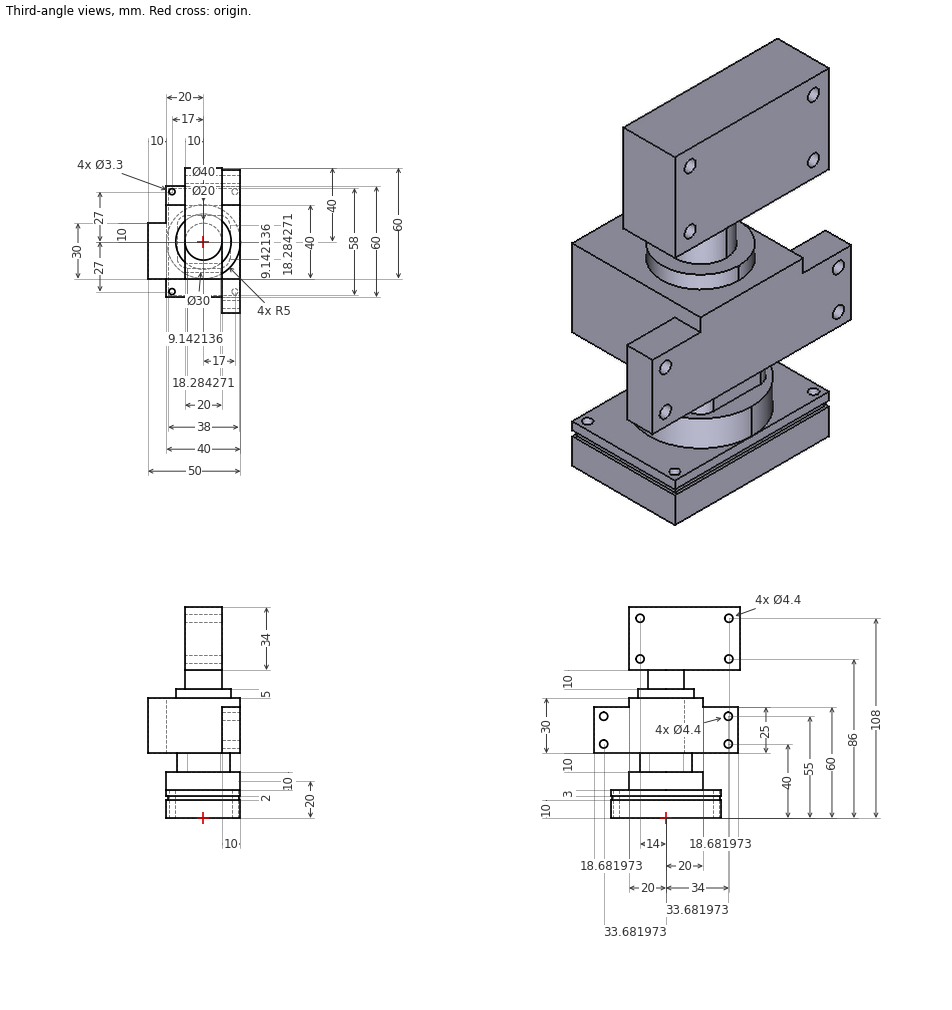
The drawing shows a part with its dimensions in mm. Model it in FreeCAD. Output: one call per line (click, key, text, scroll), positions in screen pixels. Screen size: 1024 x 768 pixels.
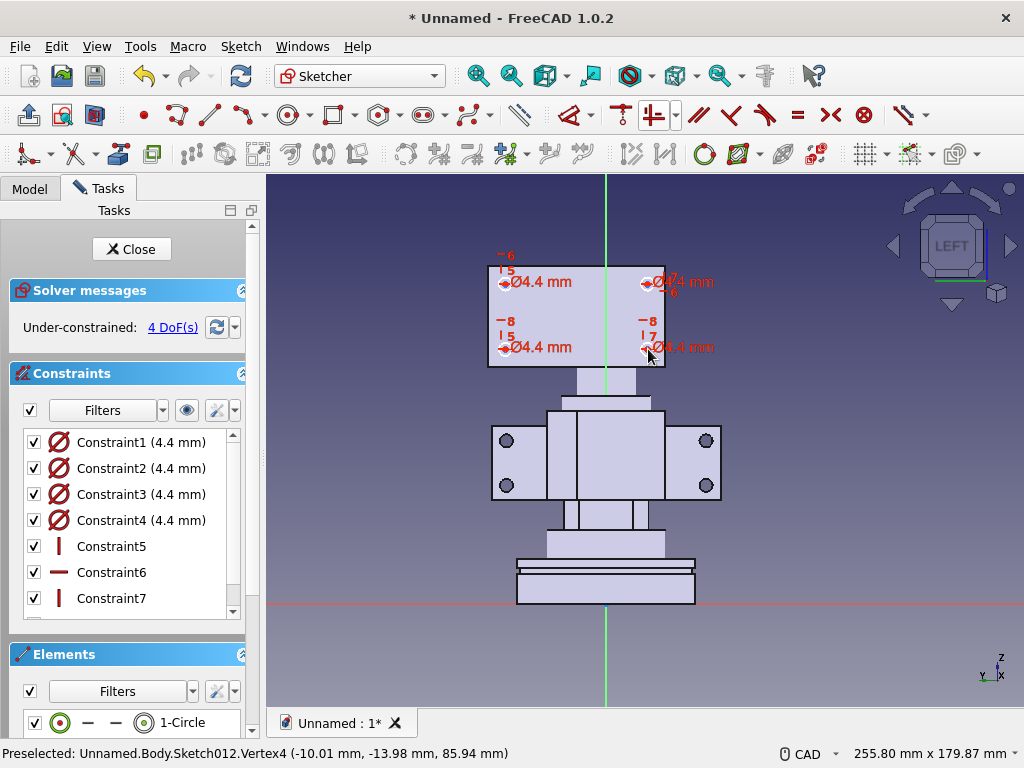
click(568, 116)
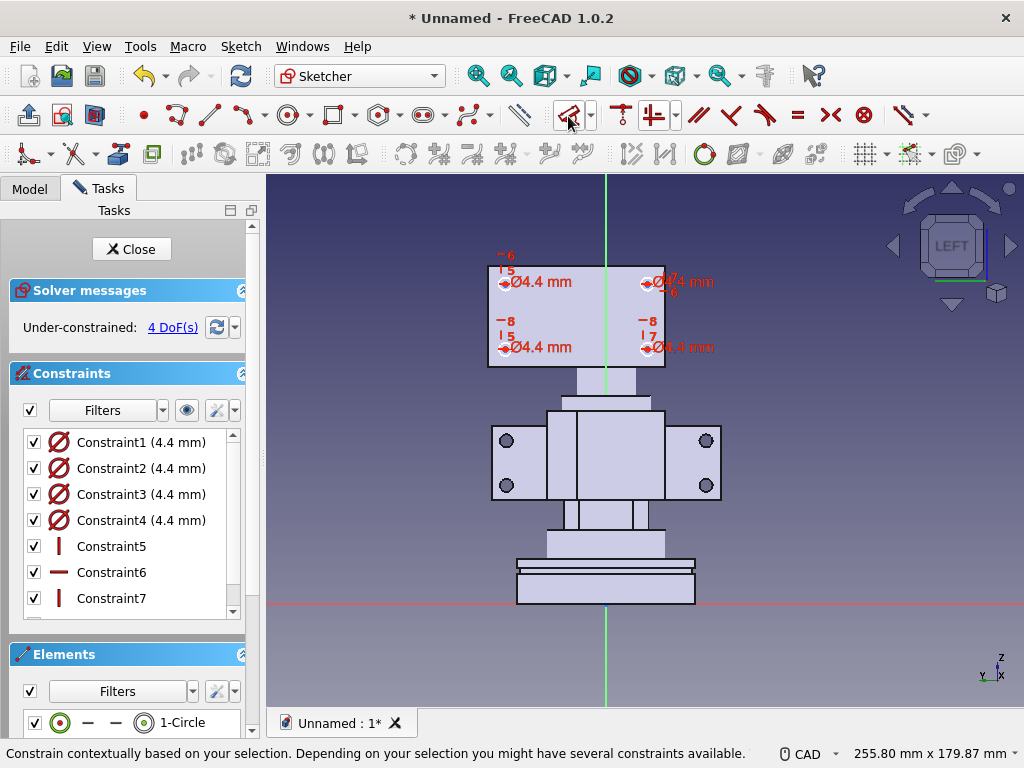
click(505, 284)
click(556, 638)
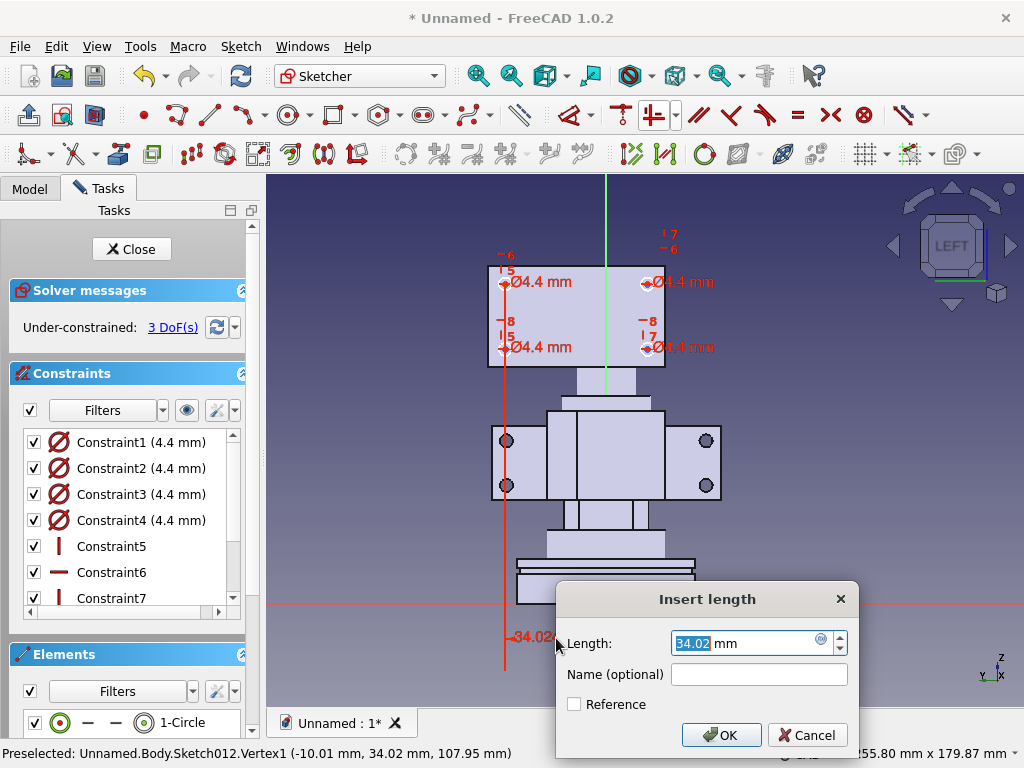
text(34)
key(Return)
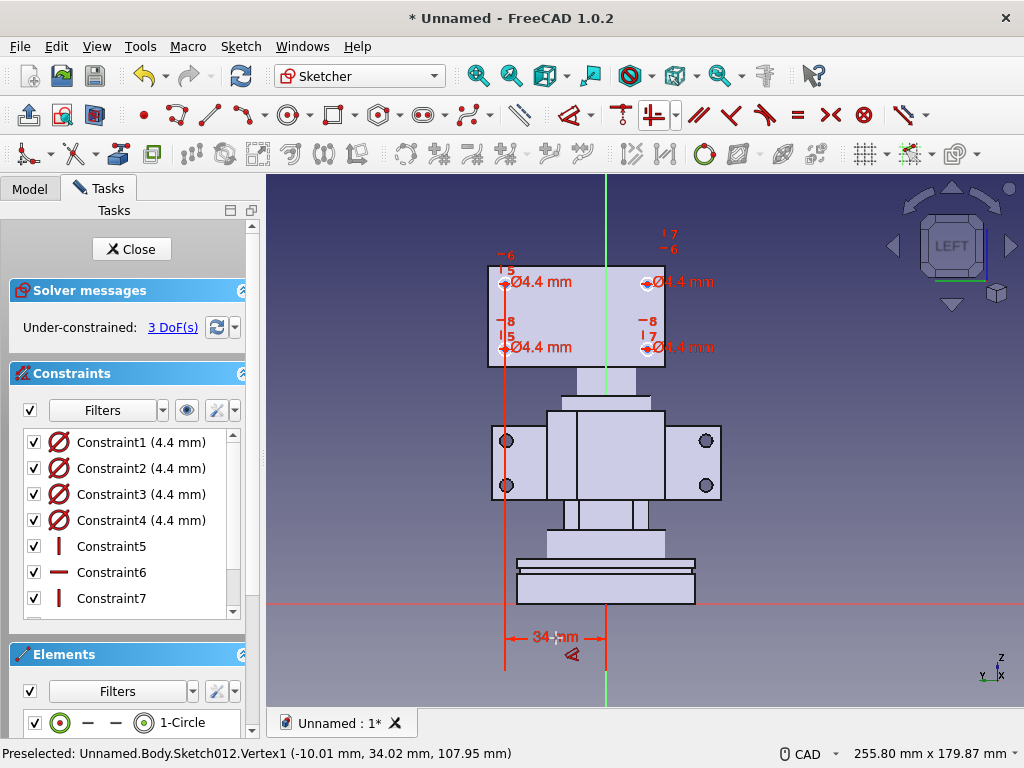
click(505, 349)
click(471, 477)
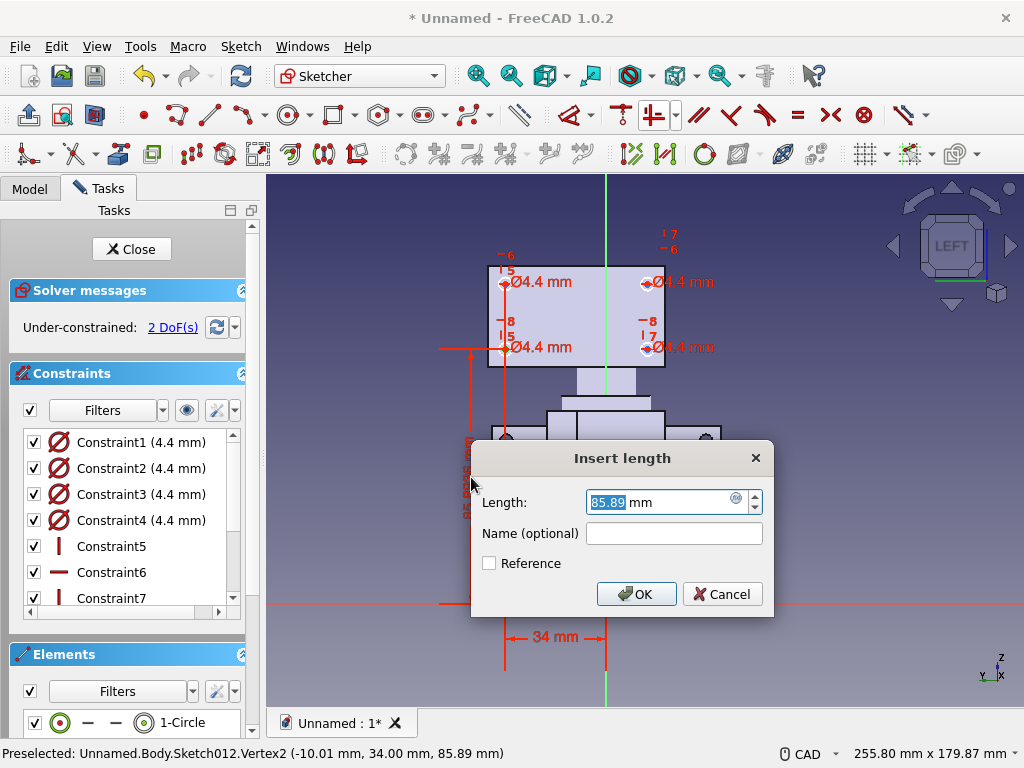
text(86)
key(Return)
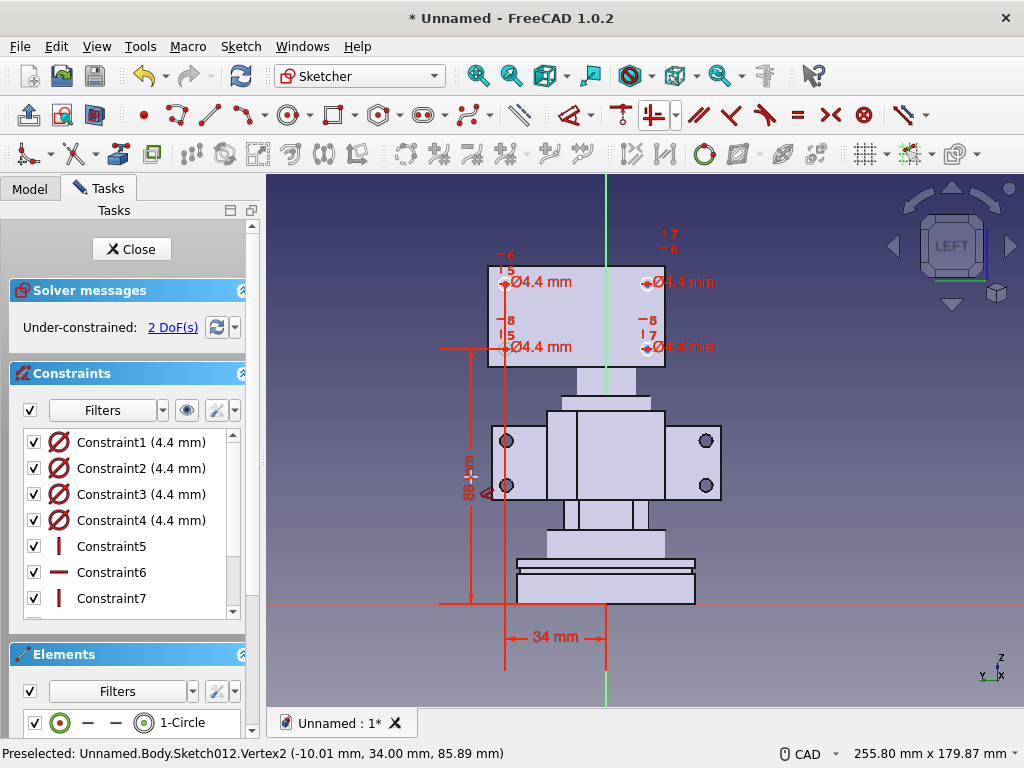
click(648, 284)
click(627, 638)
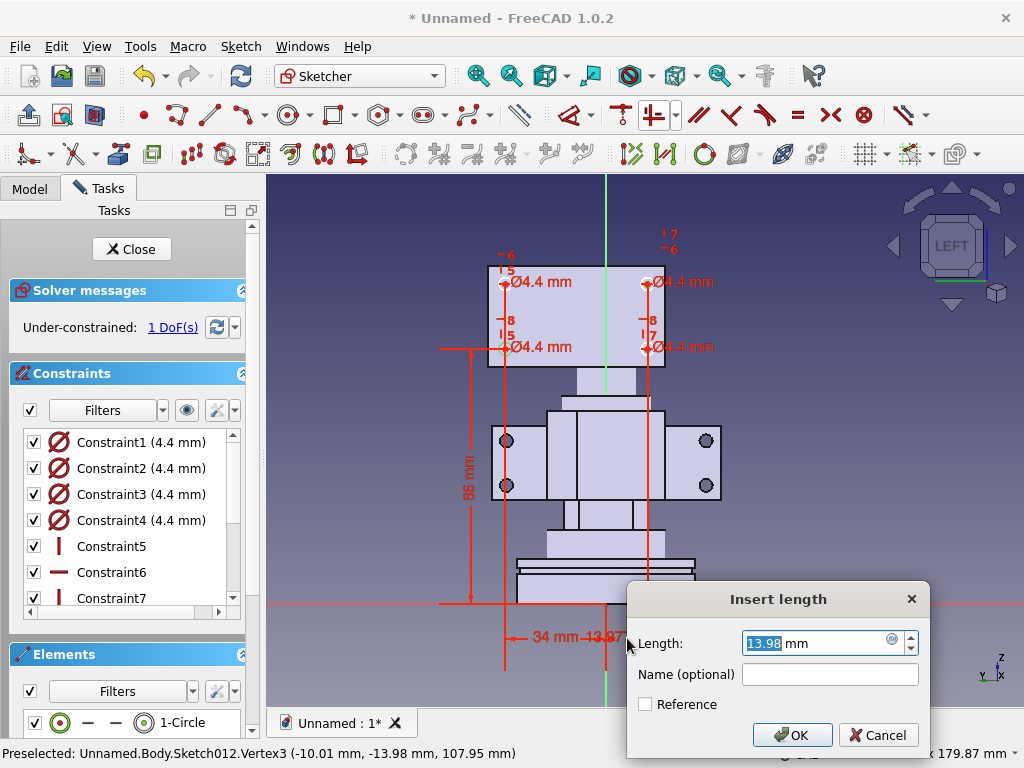
text(14)
key(Return)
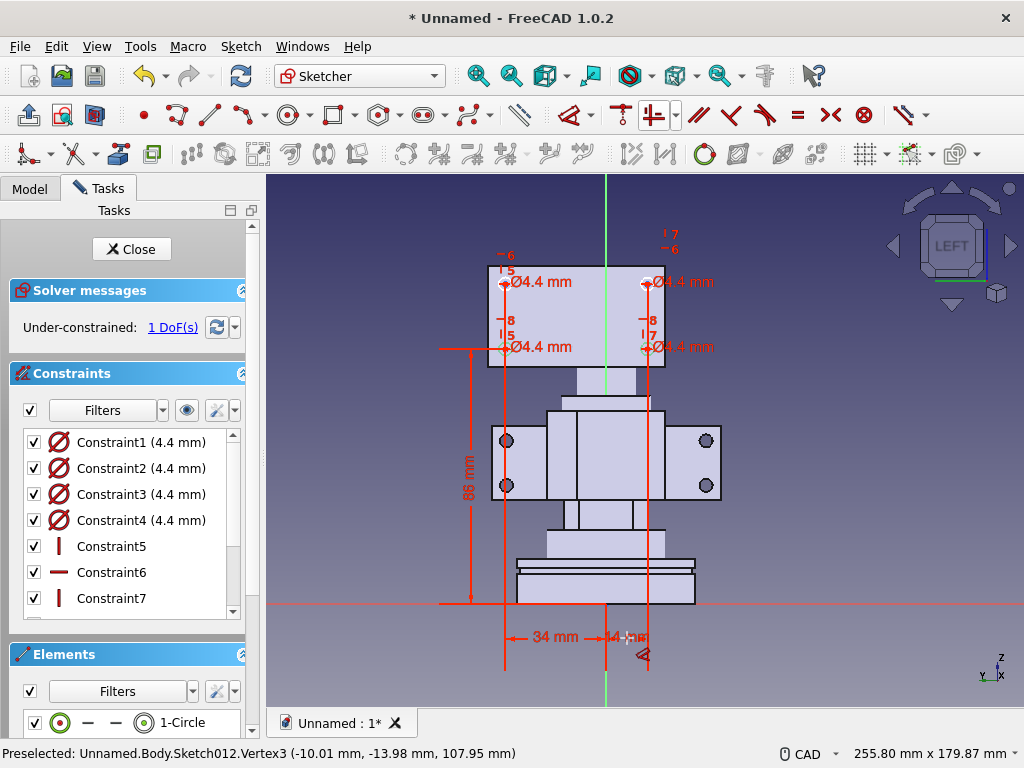
click(505, 284)
click(471, 444)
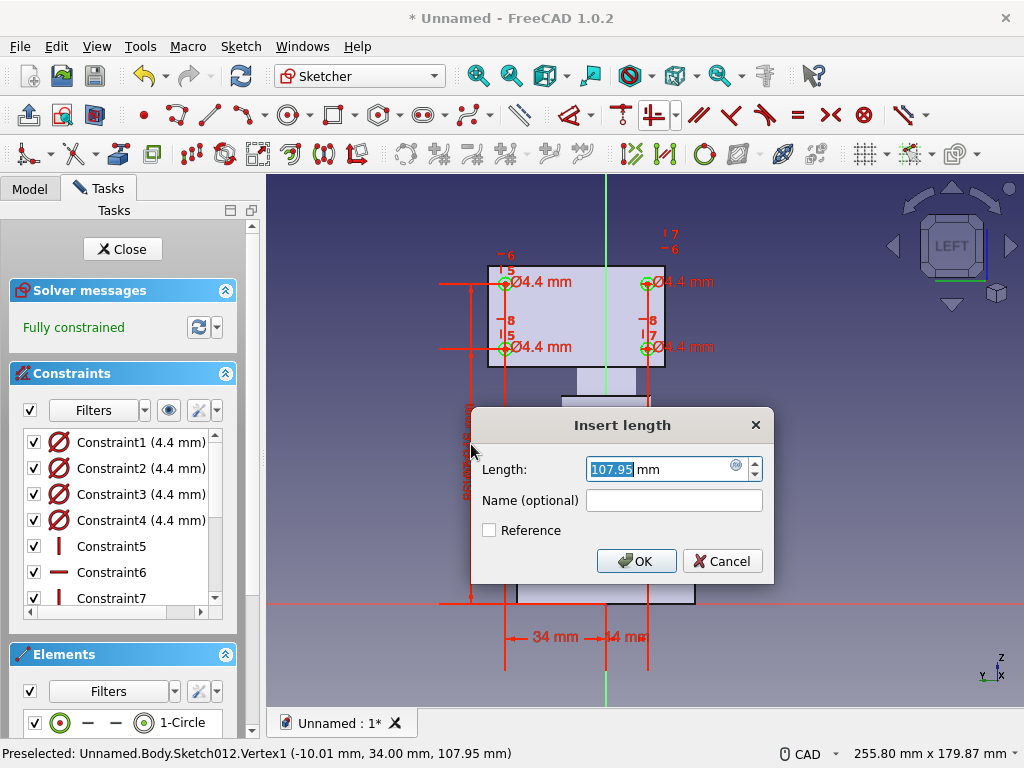
text(108)
key(Return)
key(Escape)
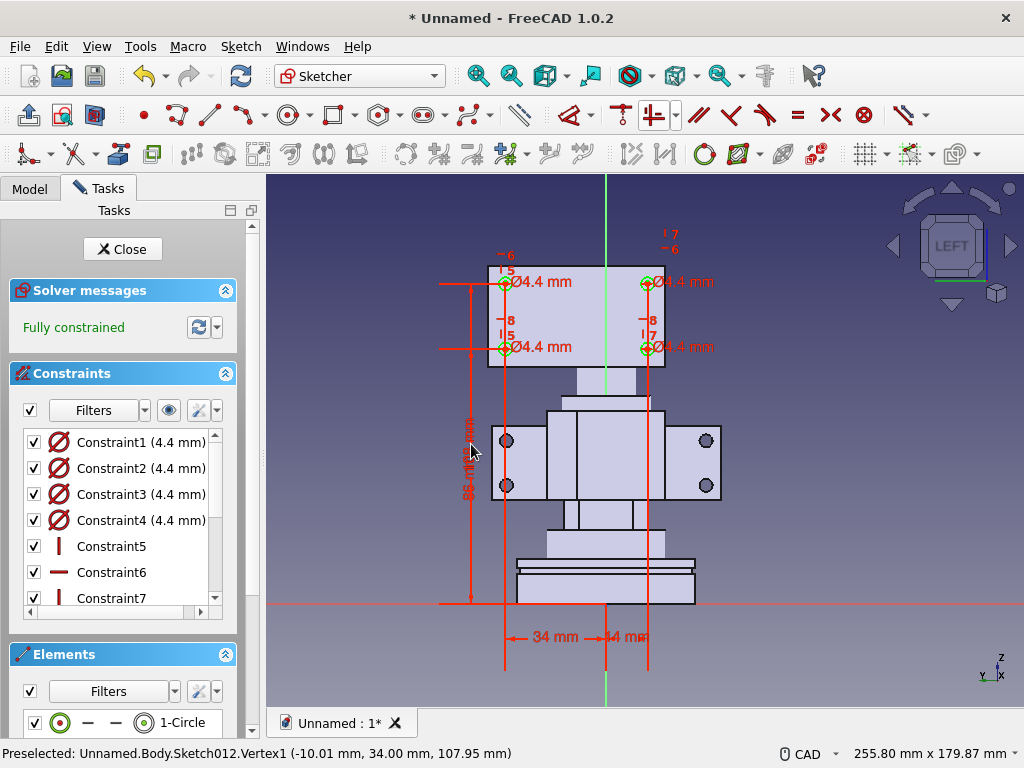
click(123, 249)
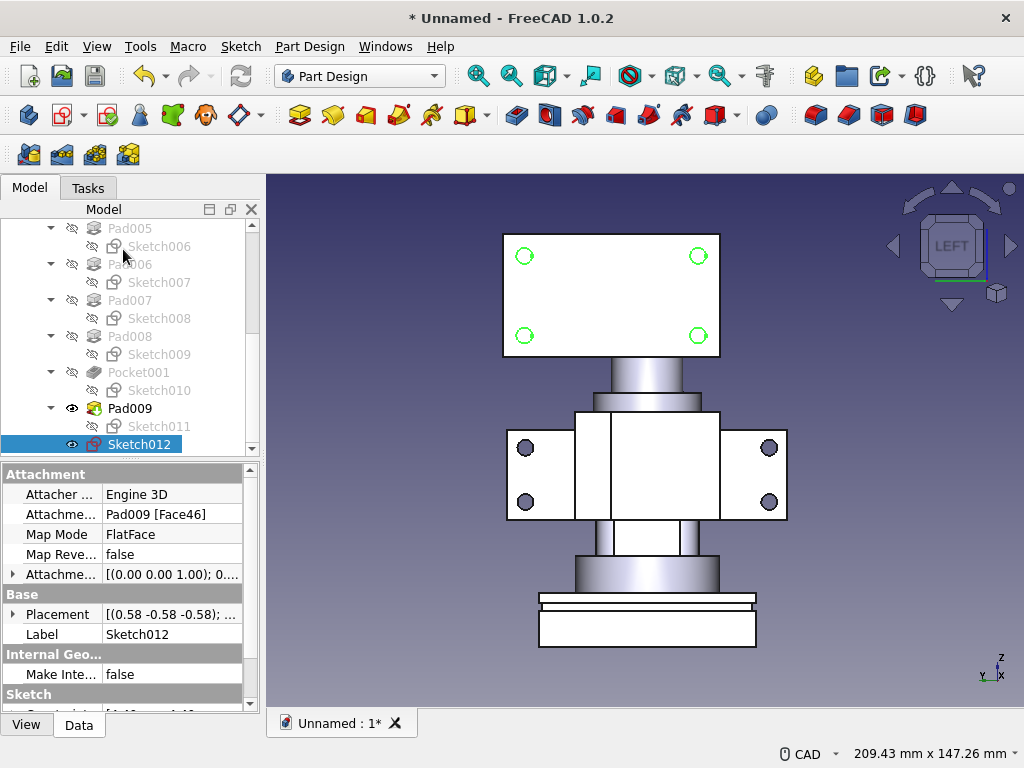
click(517, 116)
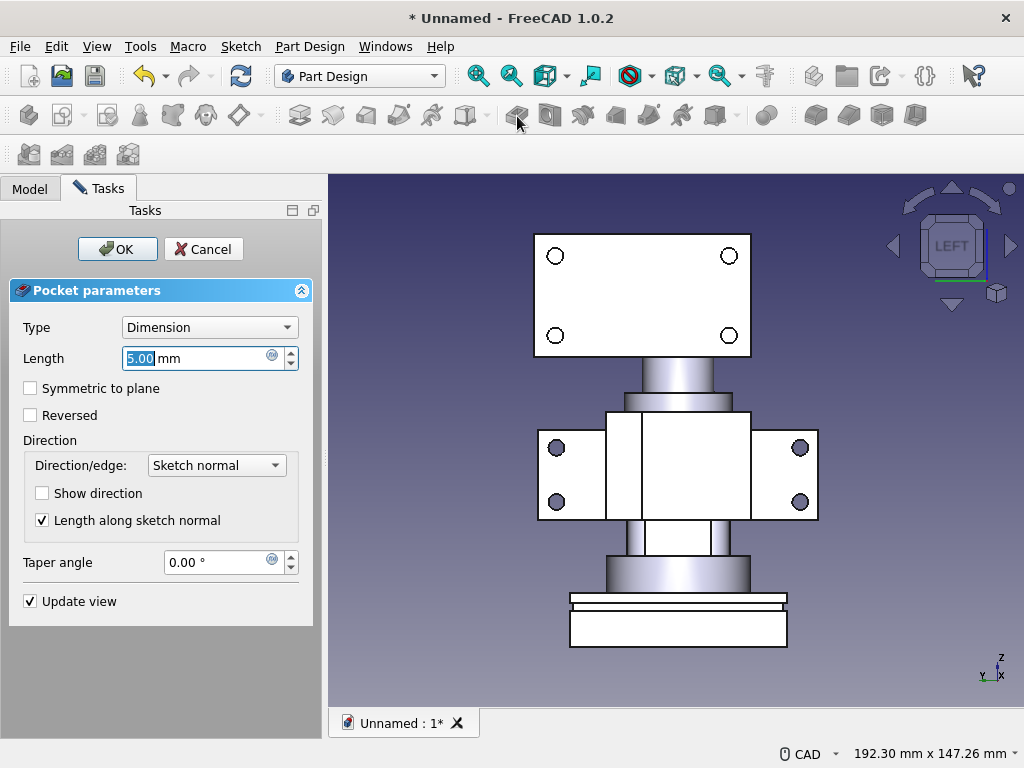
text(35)
key(Tab)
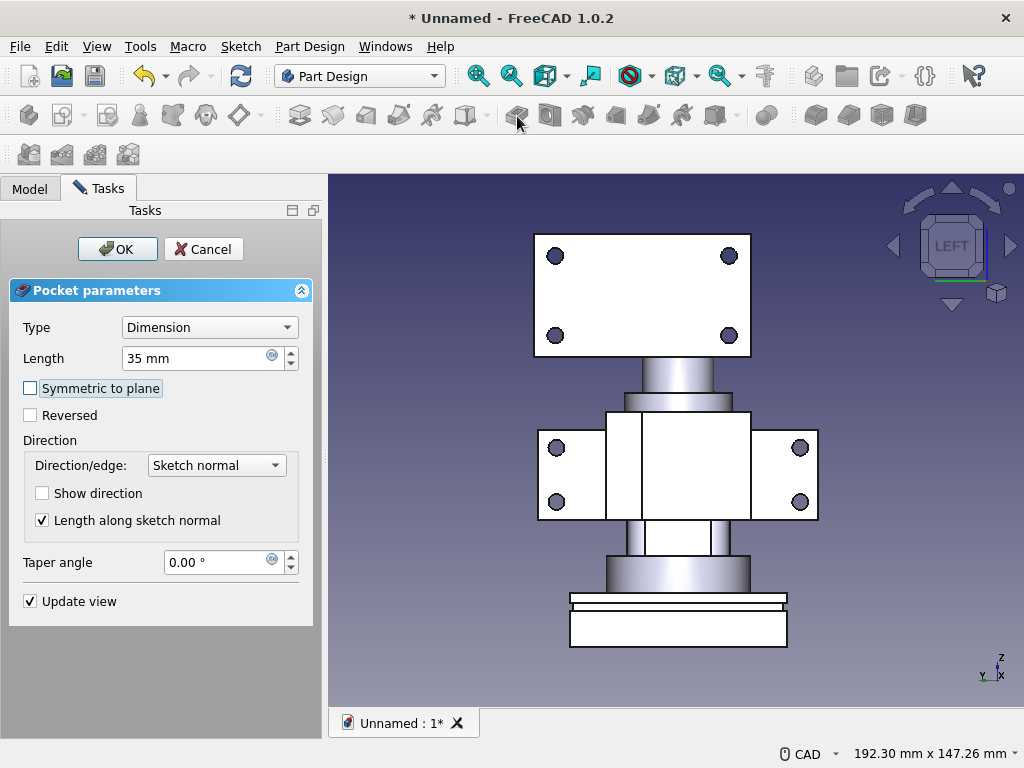
click(118, 249)